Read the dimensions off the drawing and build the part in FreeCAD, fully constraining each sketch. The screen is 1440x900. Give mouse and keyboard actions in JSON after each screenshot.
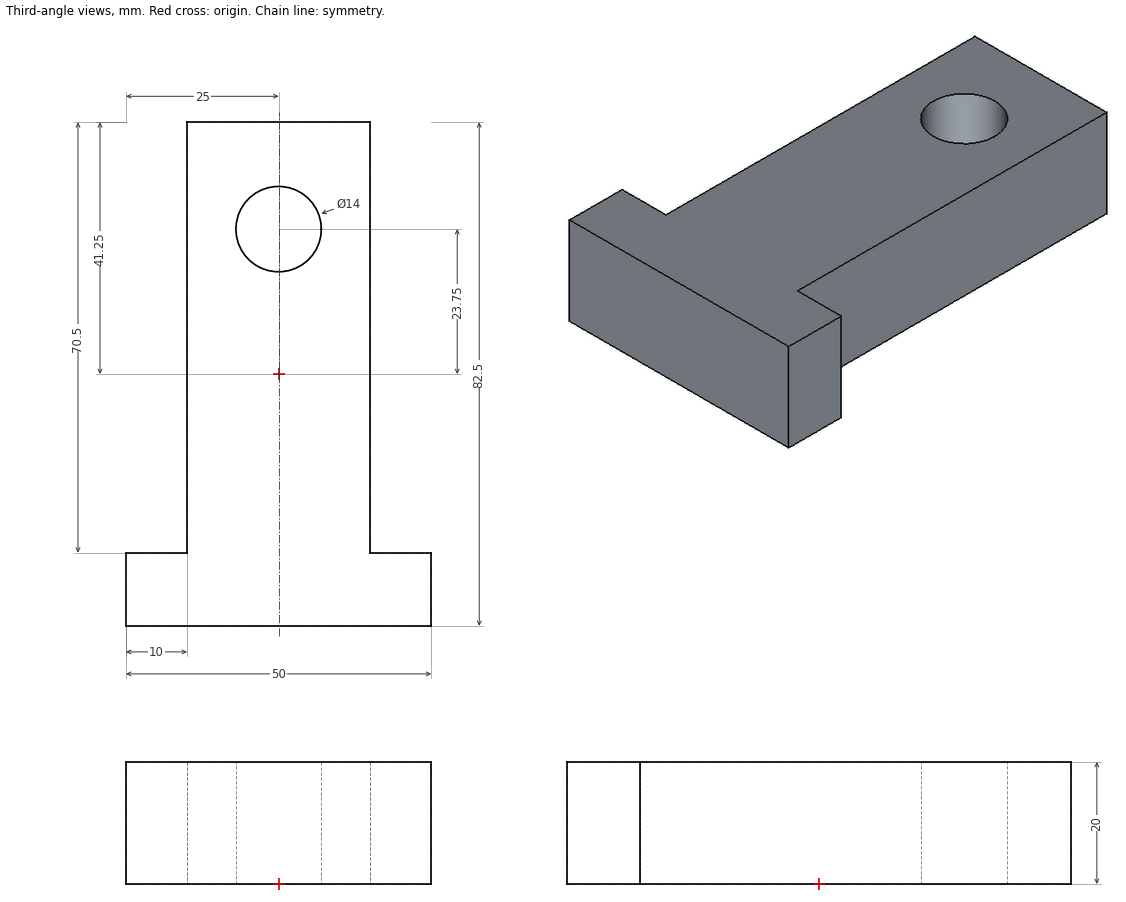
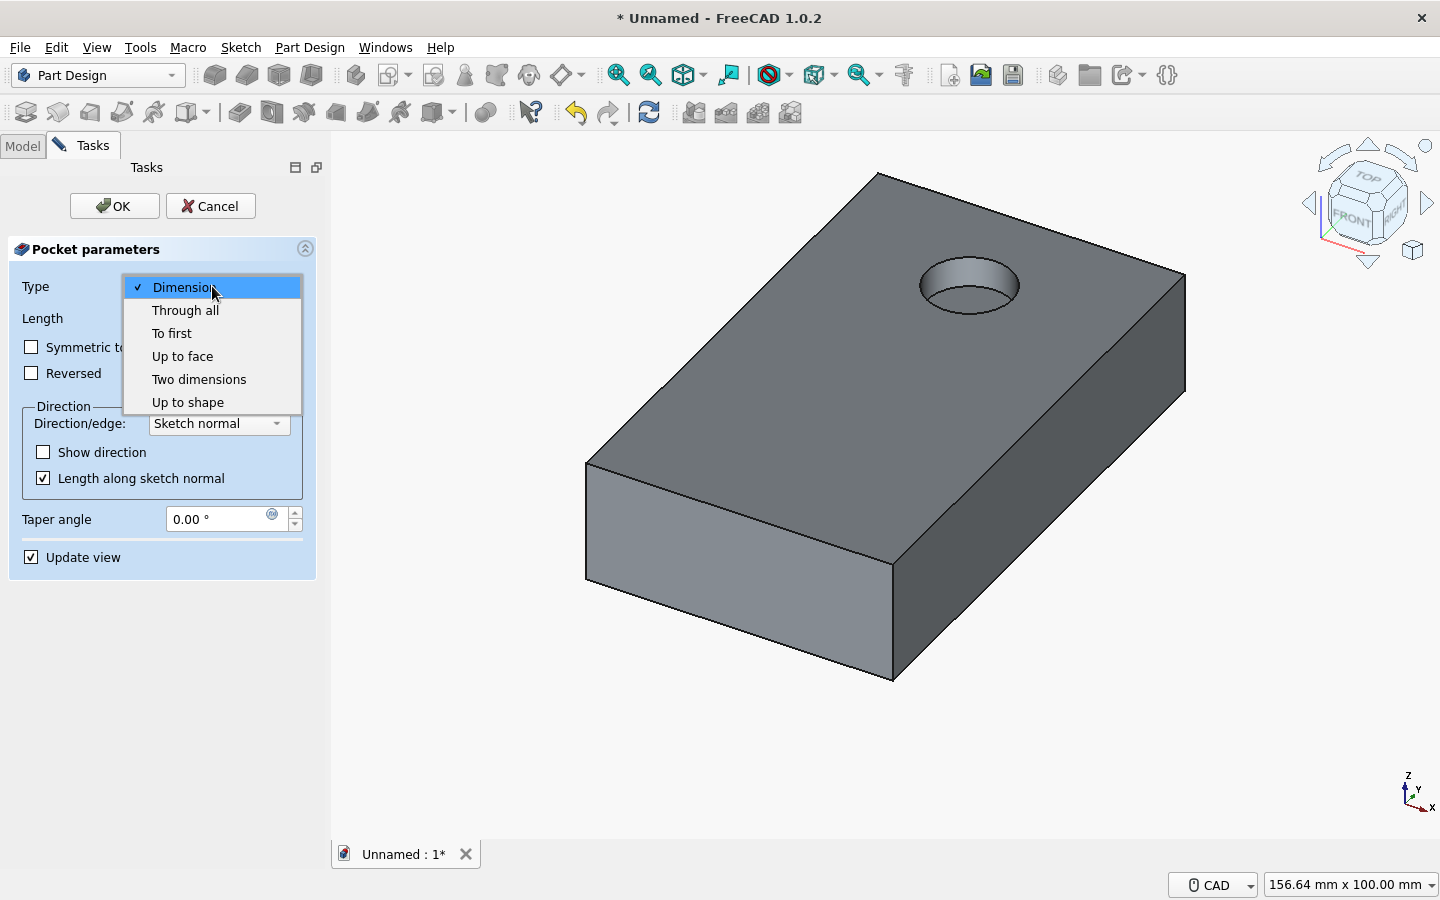
{"action": "left_click", "coordinate": [212, 310]}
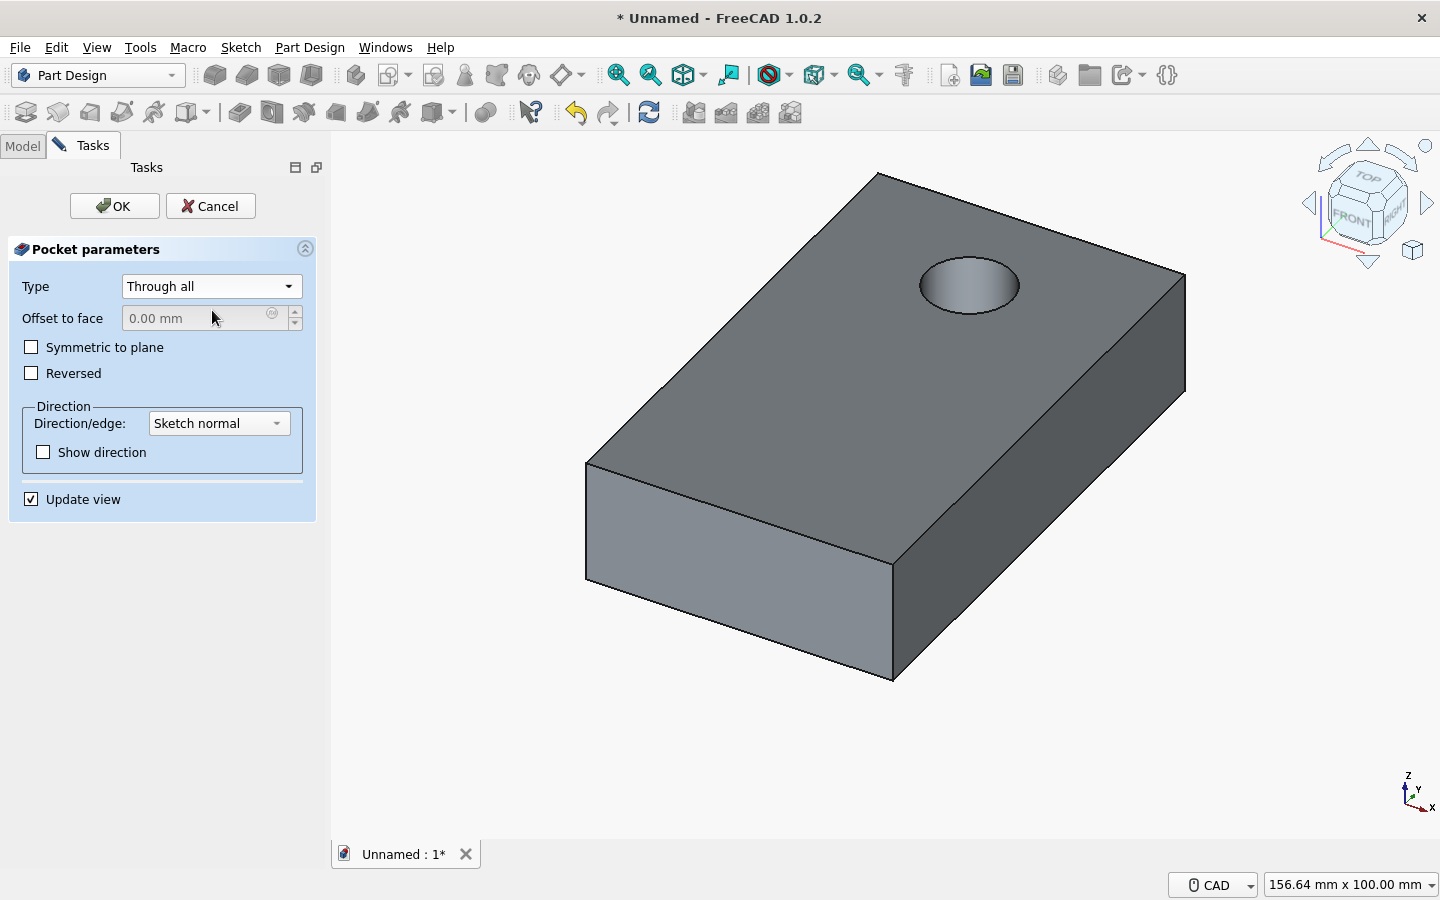
{"action": "left_click", "coordinate": [115, 206]}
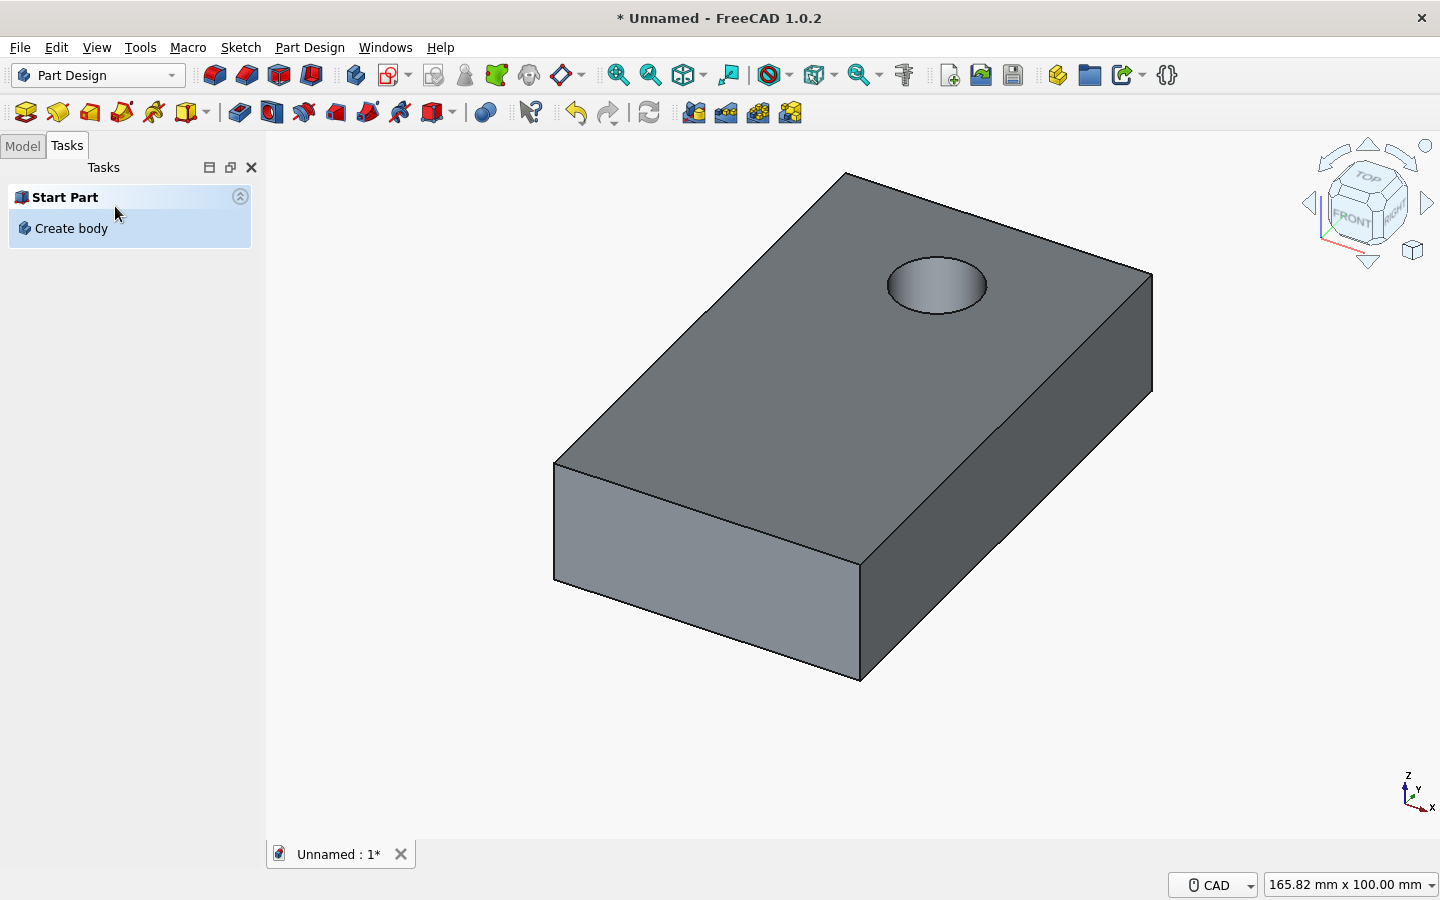
{"action": "left_click", "coordinate": [811, 409]}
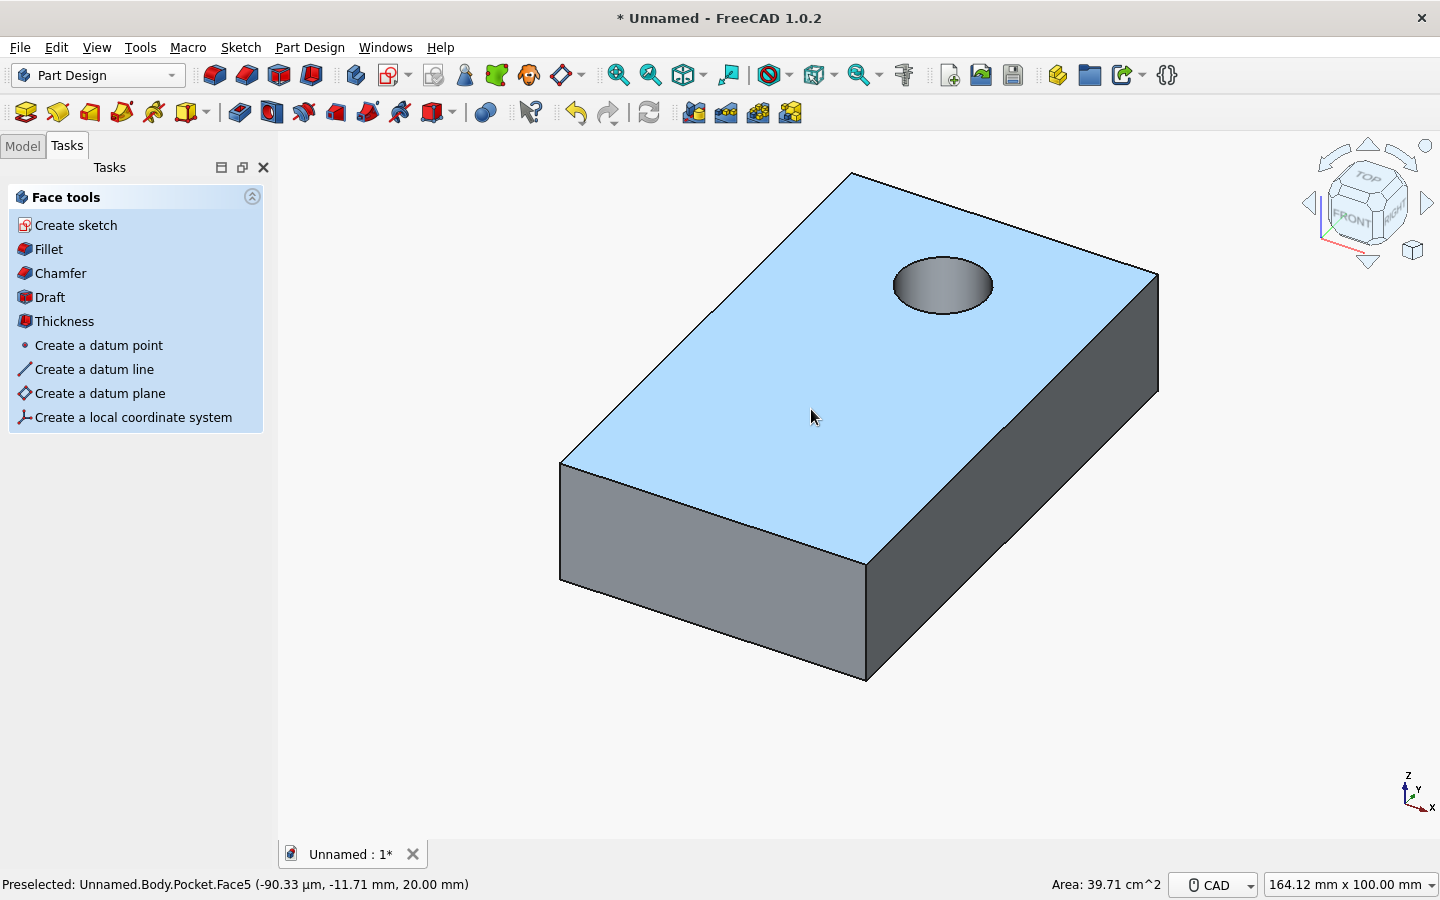
{"action": "left_click", "coordinate": [388, 76]}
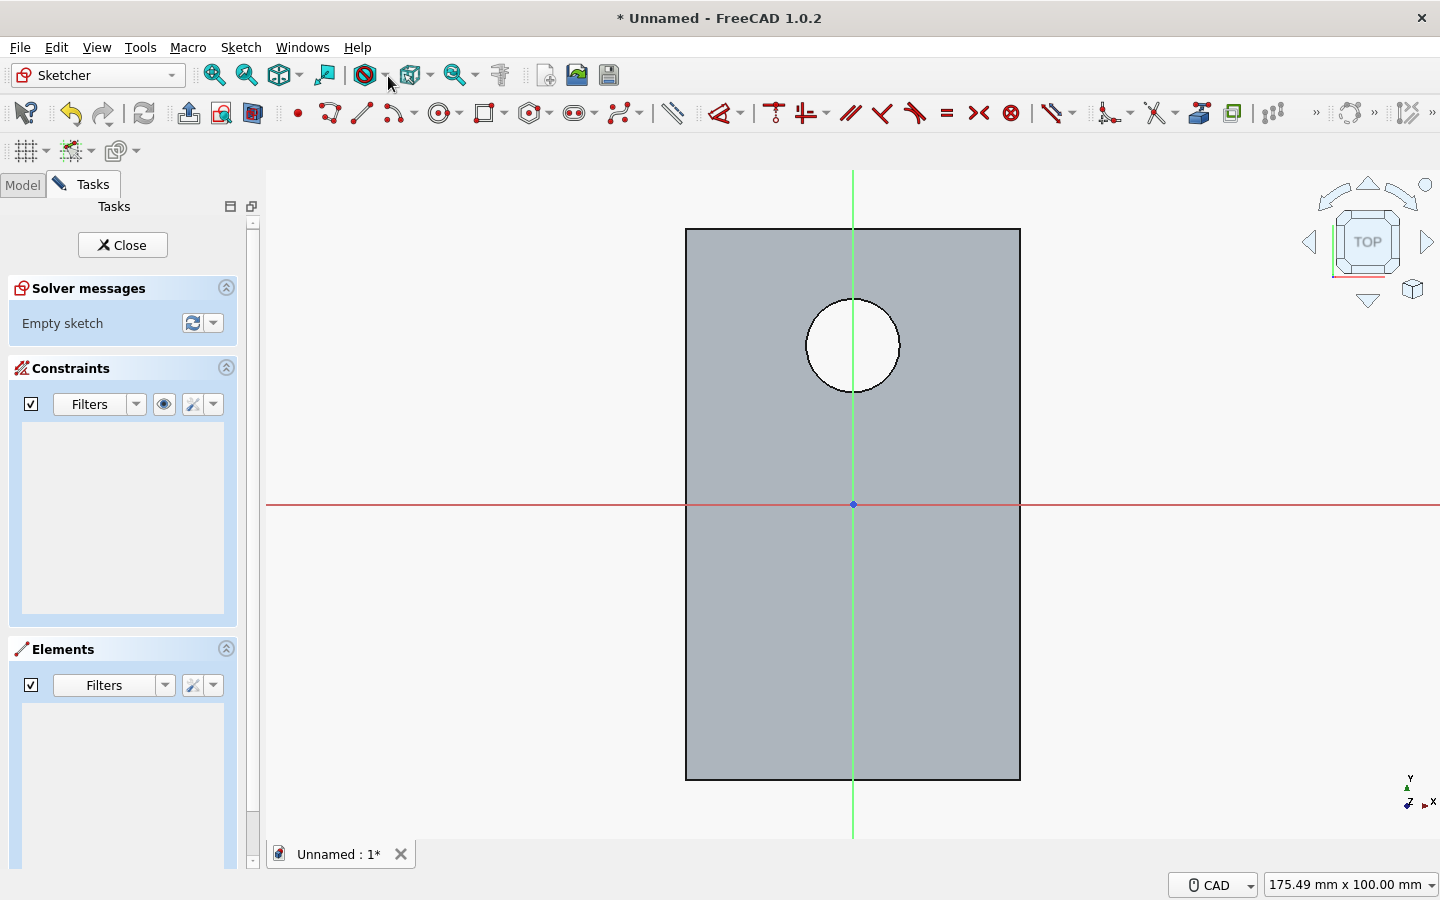
{"action": "left_click", "coordinate": [484, 114]}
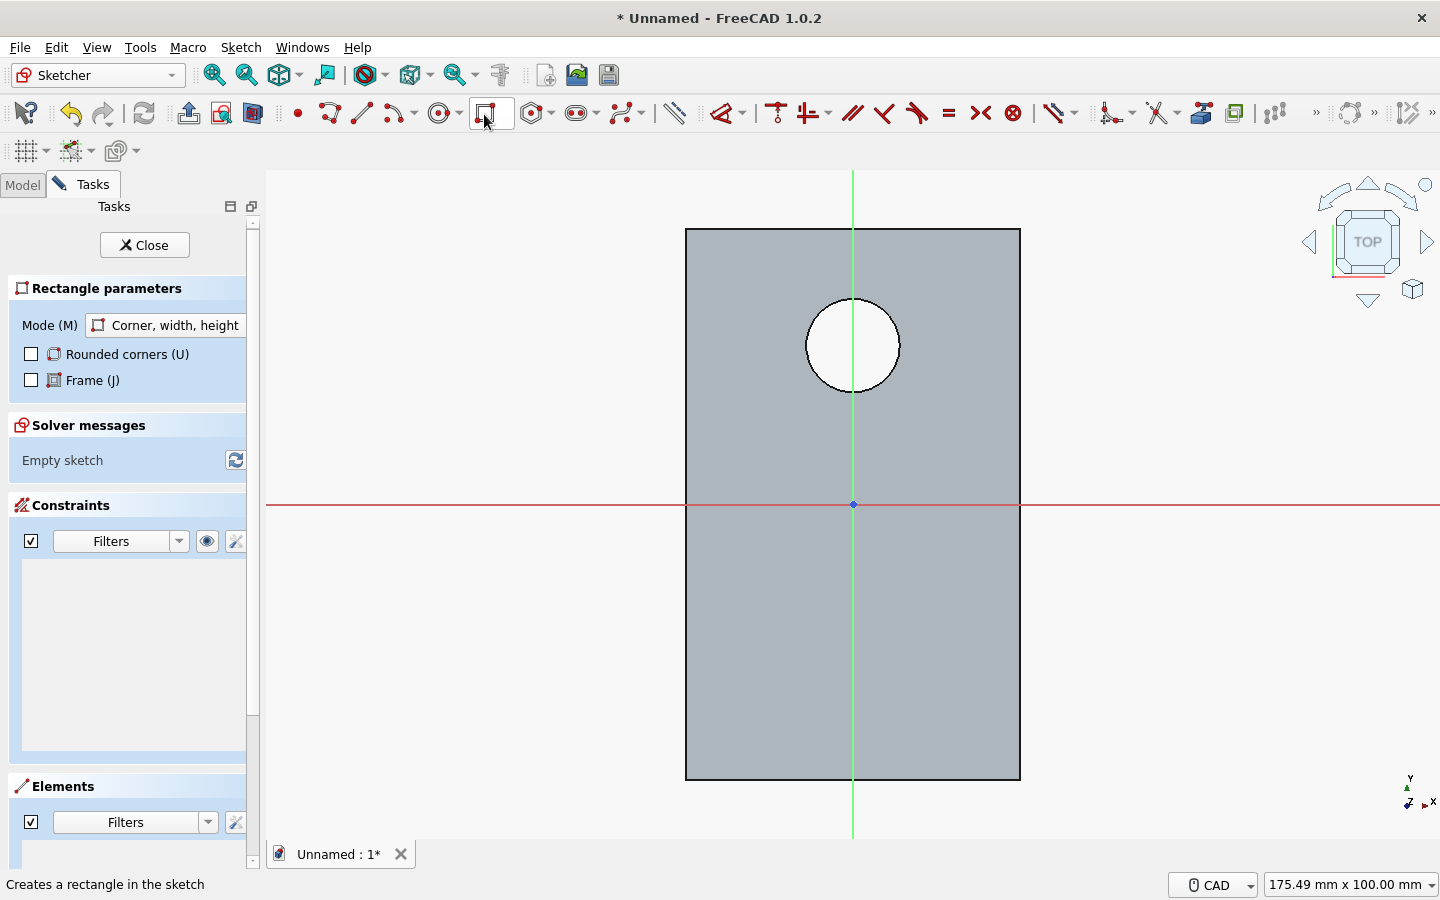
{"action": "left_click", "coordinate": [686, 229]}
{"action": "left_click", "coordinate": [753, 700]}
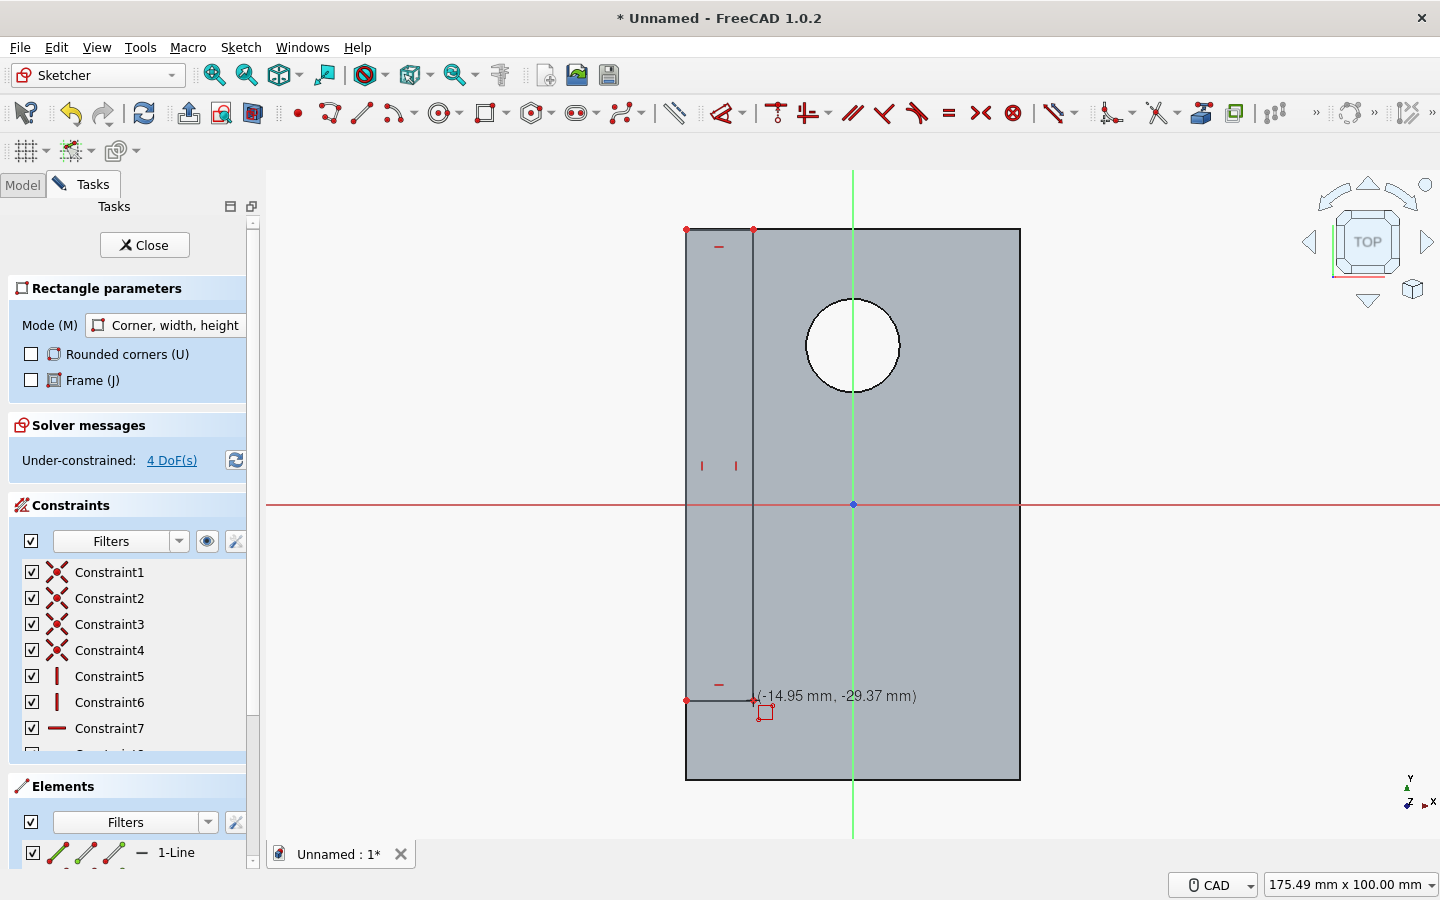
{"action": "left_click", "coordinate": [953, 229]}
{"action": "left_click", "coordinate": [1020, 700]}
{"action": "key", "text": "Escape"}